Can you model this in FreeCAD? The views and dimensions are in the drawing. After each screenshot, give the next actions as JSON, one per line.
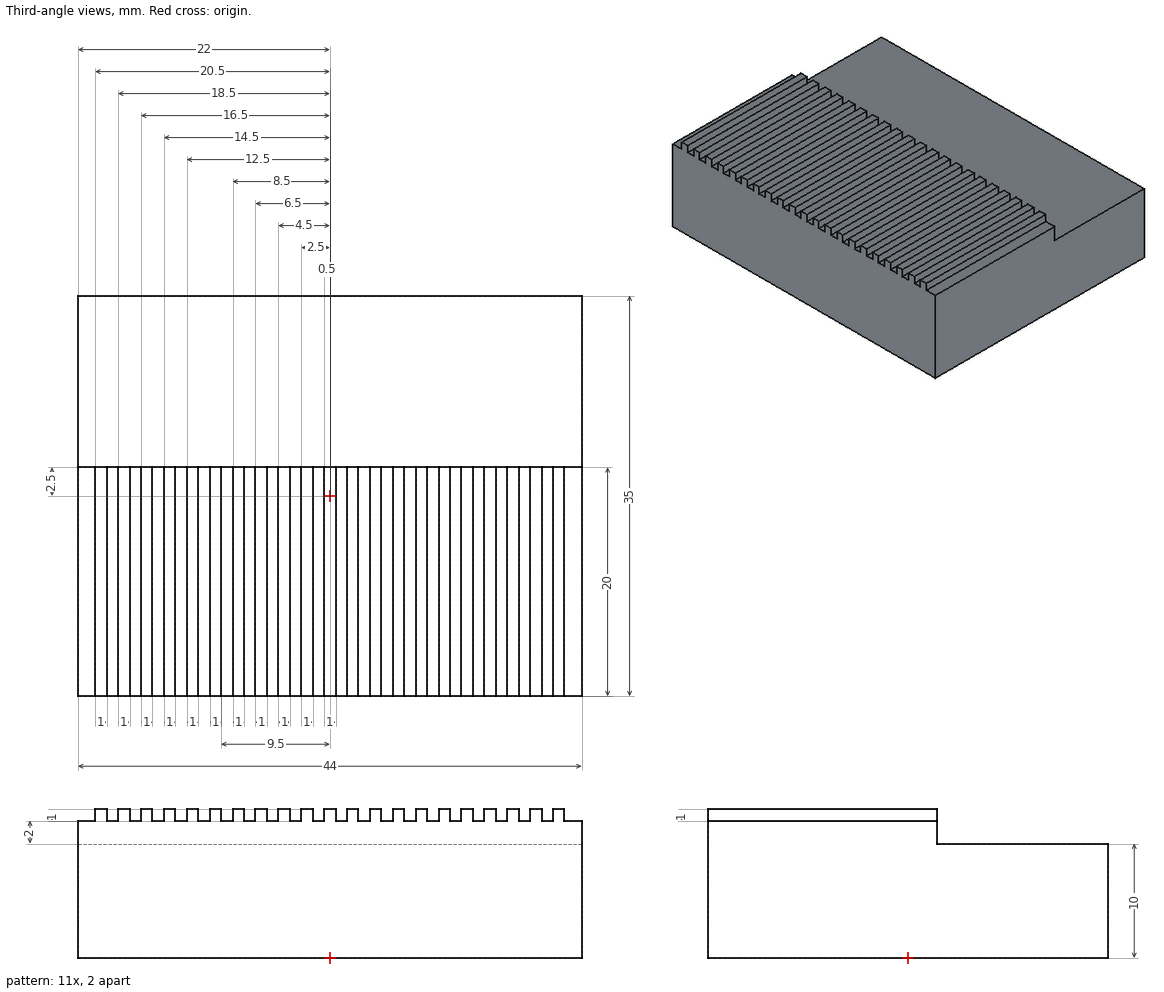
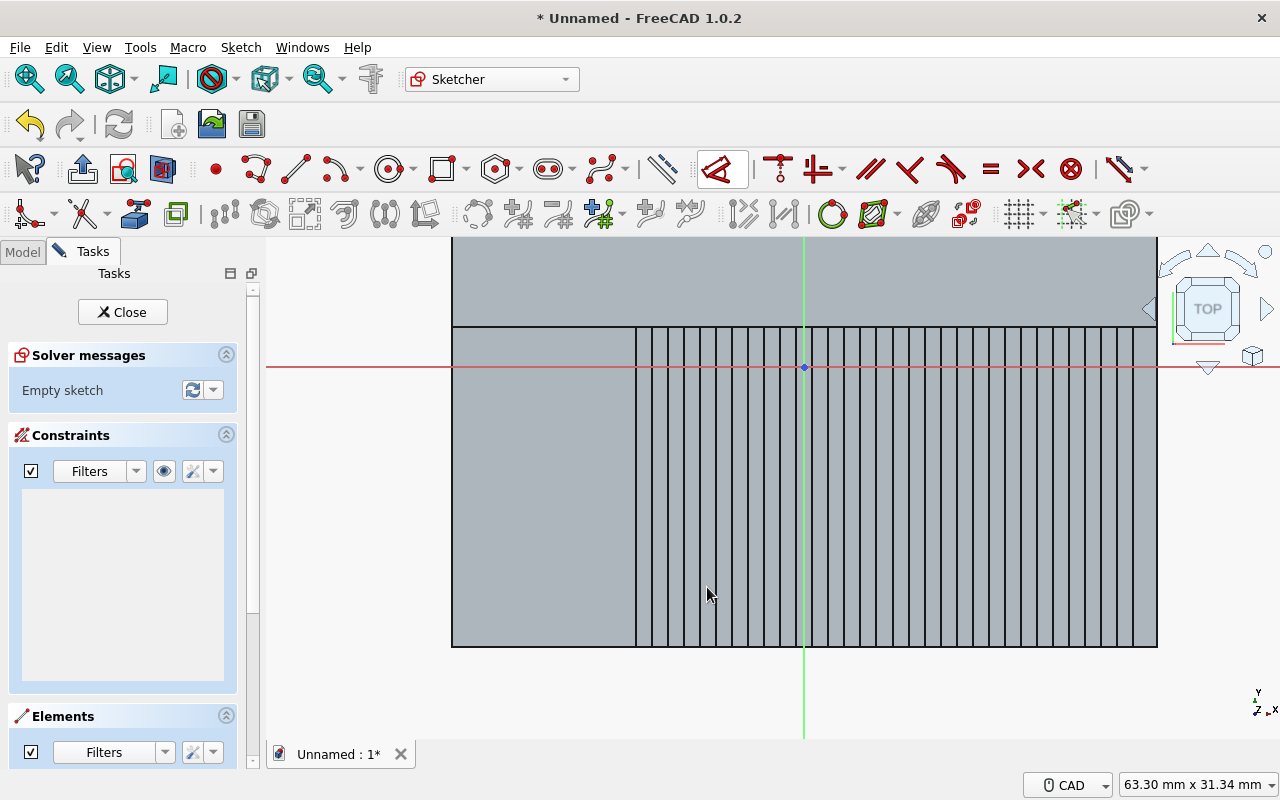
{"action": "left_click", "coordinate": [442, 170]}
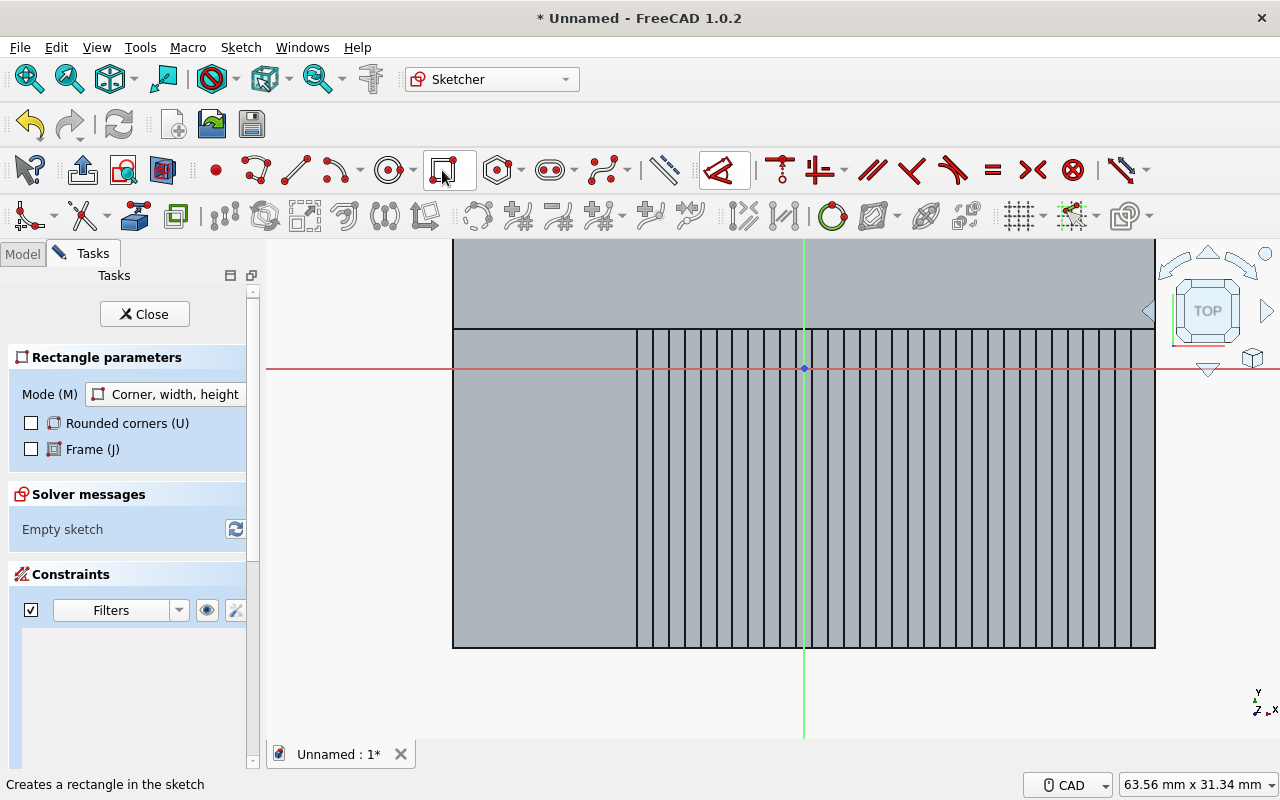
{"action": "left_click", "coordinate": [605, 329]}
{"action": "mouse_move", "coordinate": [621, 648]}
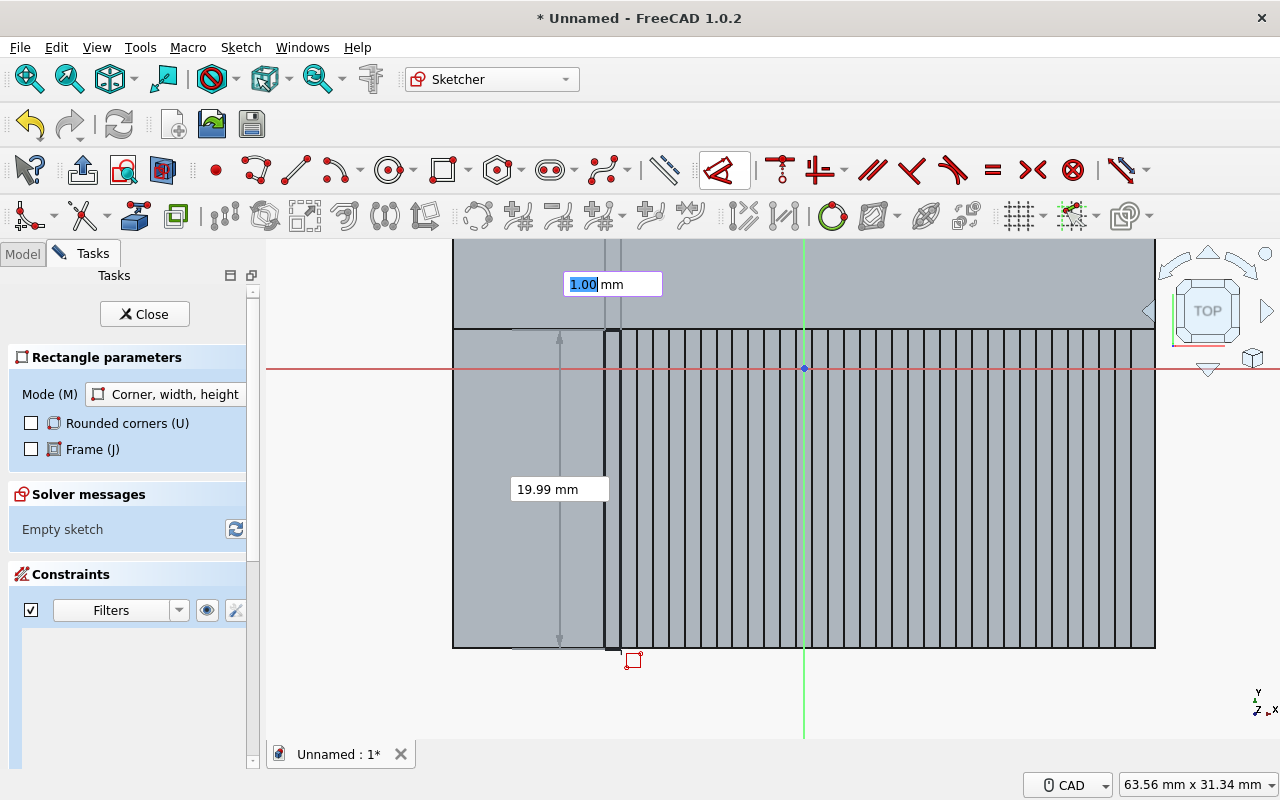
{"action": "type", "text": "1"}
{"action": "key", "text": "Tab"}
{"action": "type", "text": "20"}
{"action": "key", "text": "Return"}
{"action": "key", "text": "Escape"}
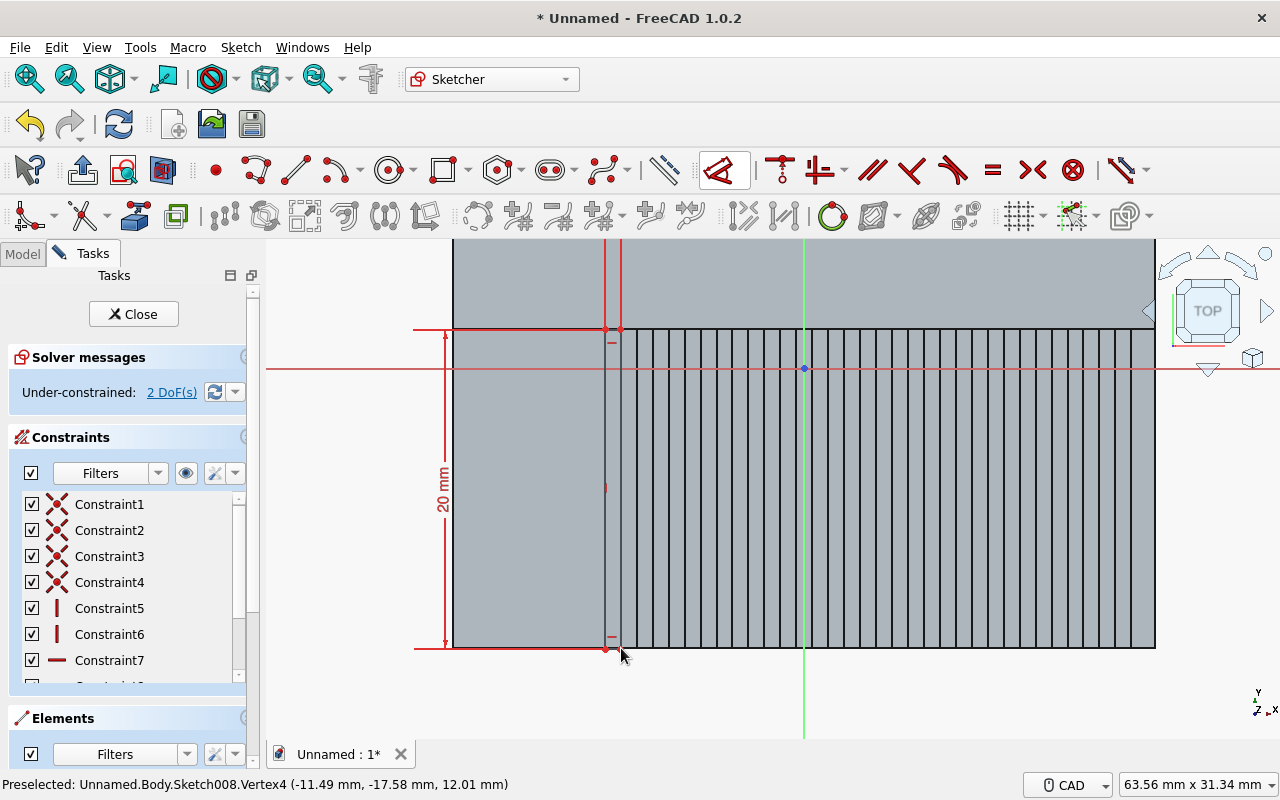
{"action": "left_click", "coordinate": [605, 330]}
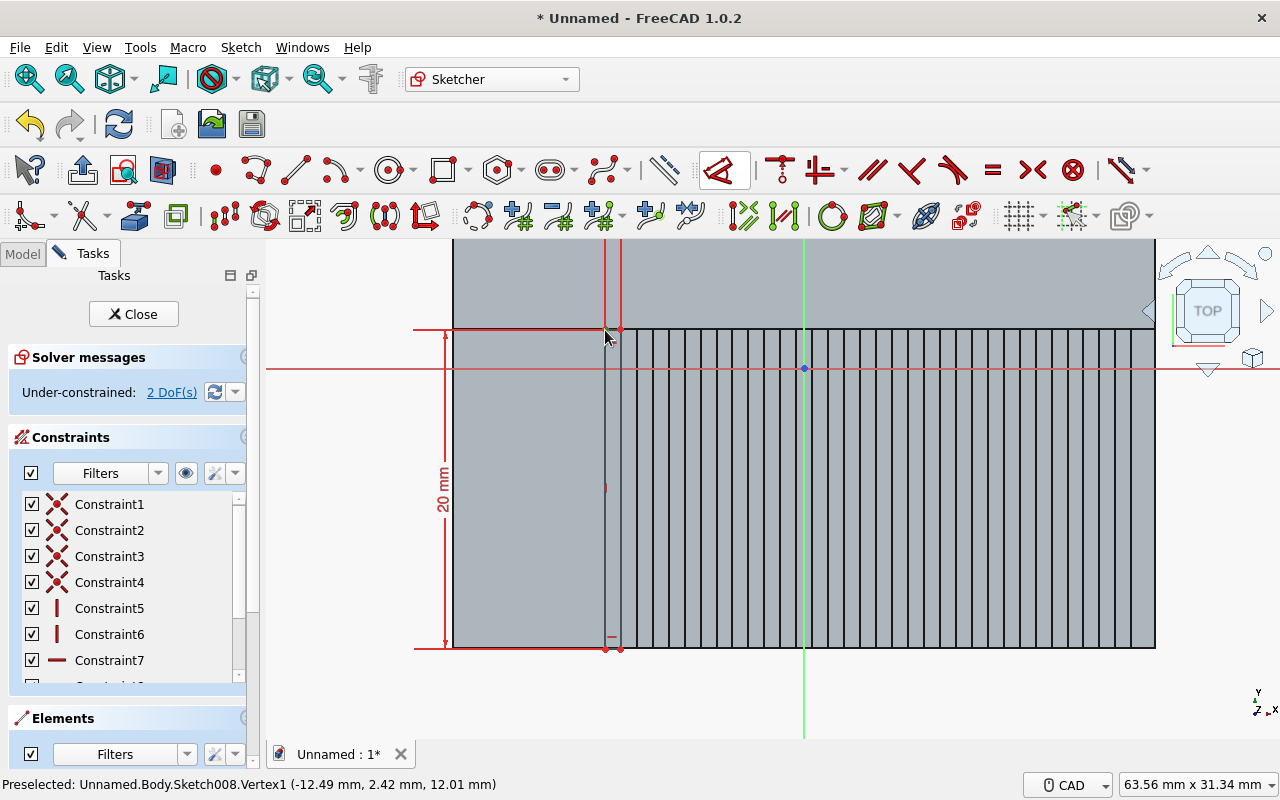
{"action": "key", "text": "i"}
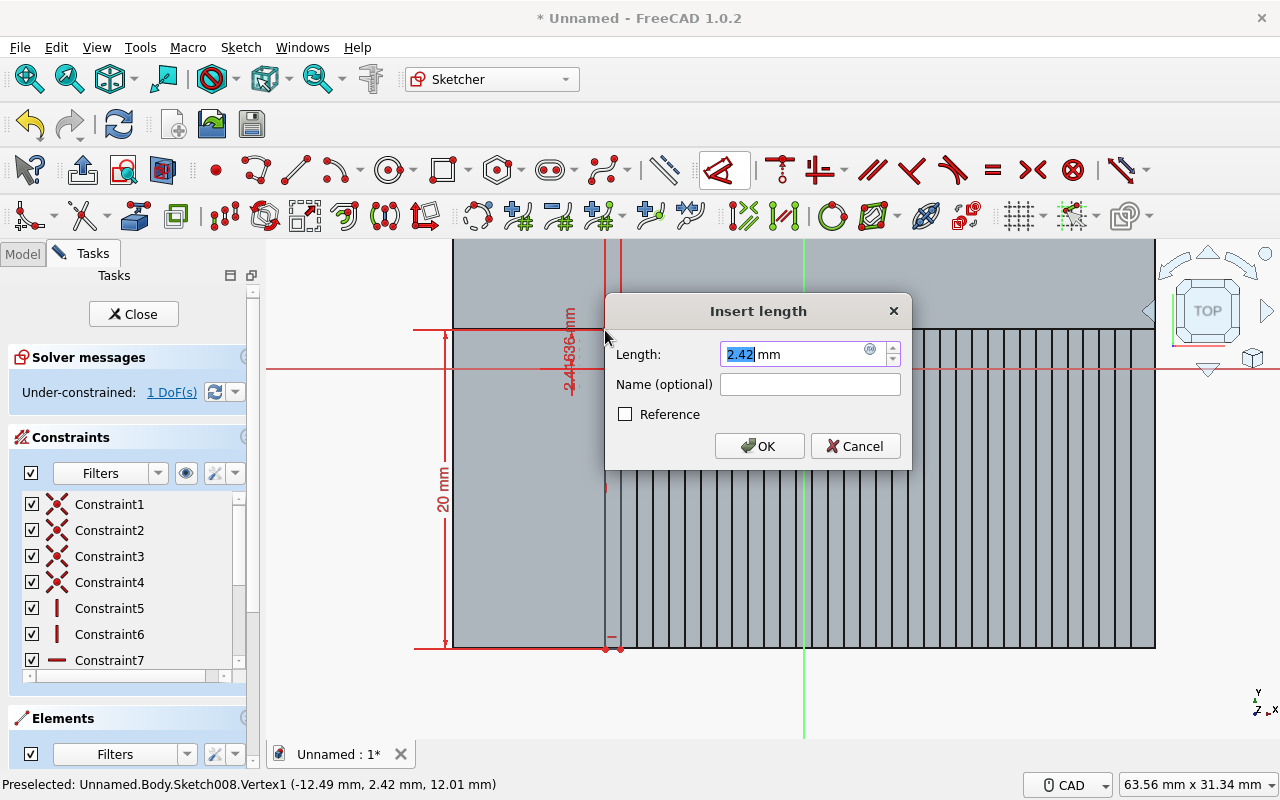
{"action": "type", "text": "2.5"}
{"action": "key", "text": "Return"}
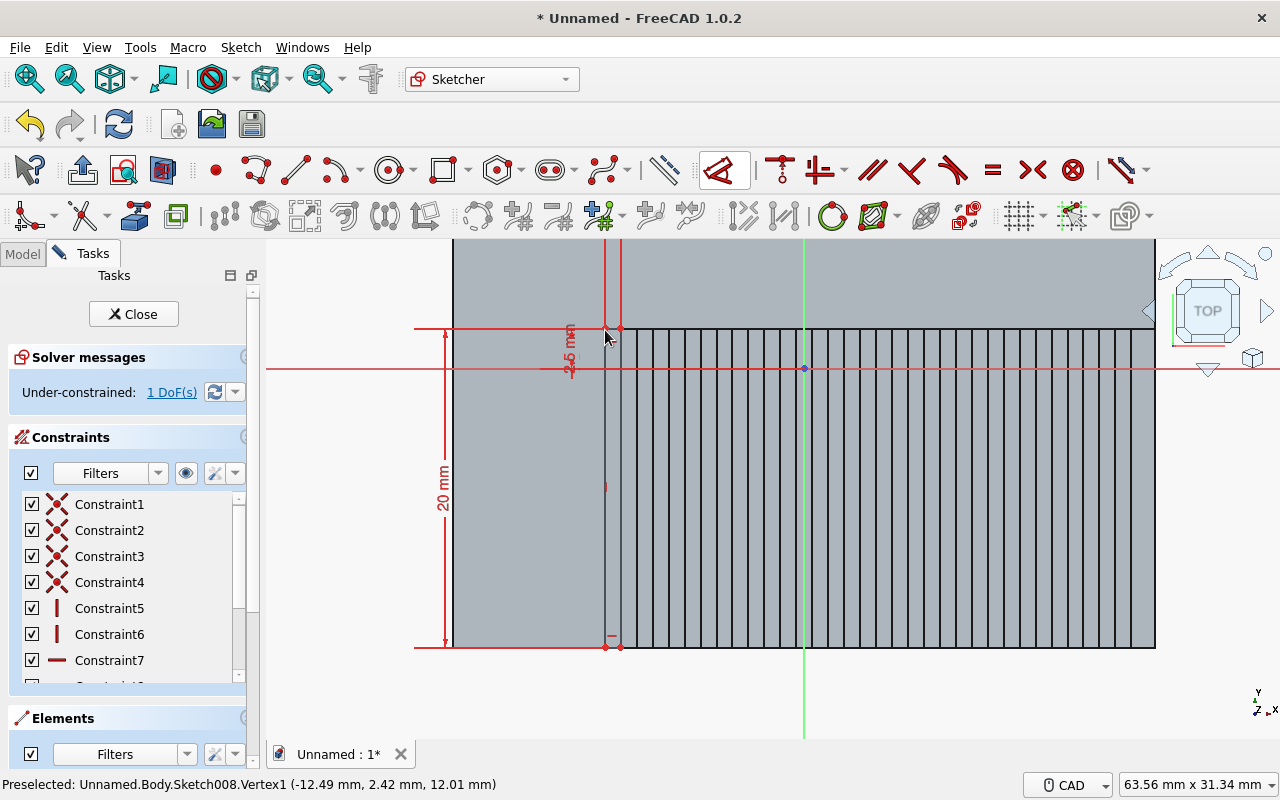
{"action": "left_click", "coordinate": [605, 329]}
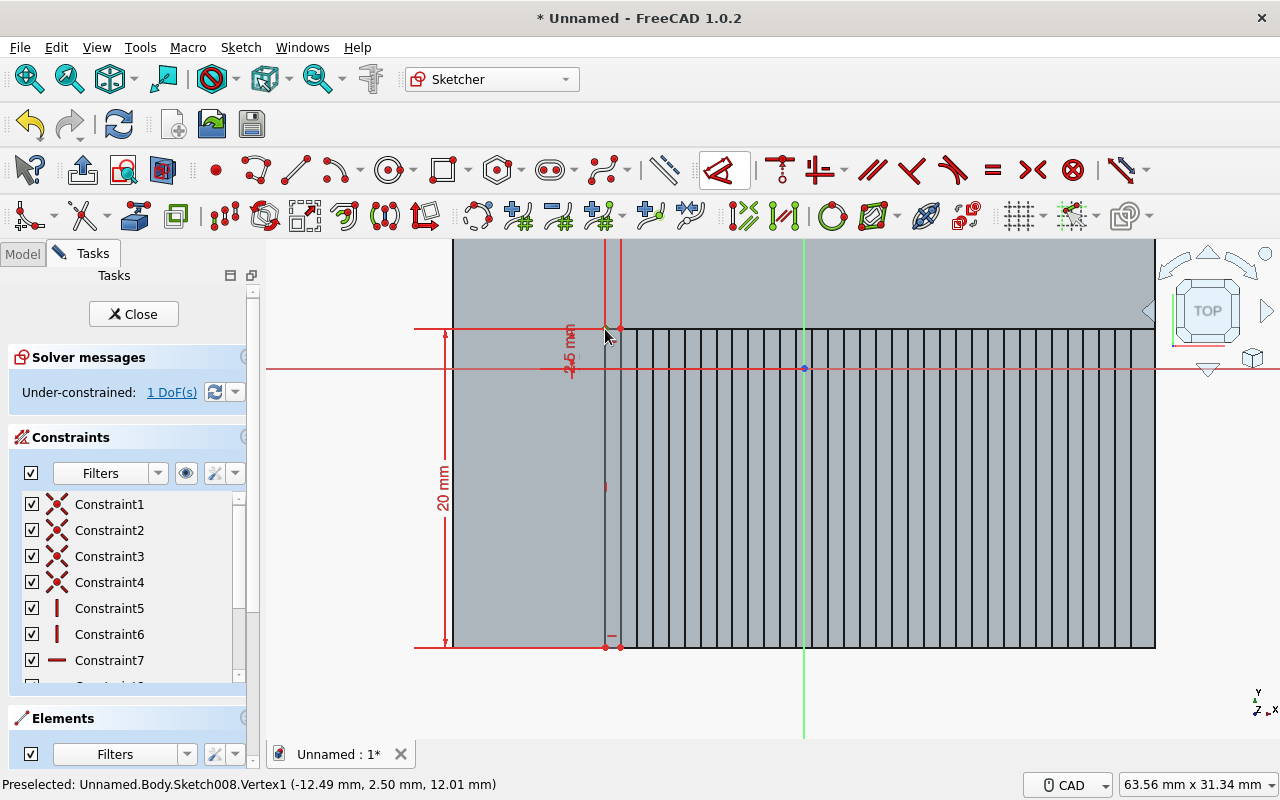
{"action": "left_click", "coordinate": [744, 170]}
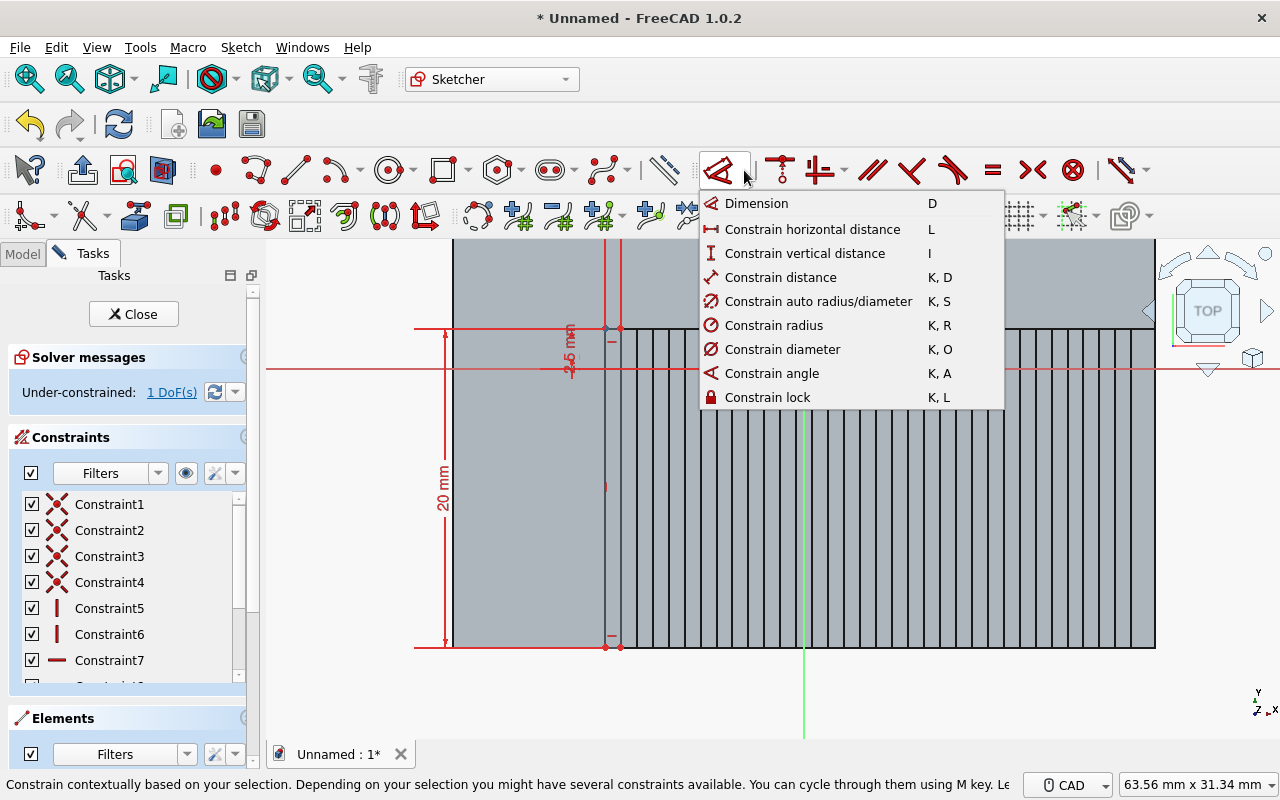
{"action": "left_click", "coordinate": [852, 229]}